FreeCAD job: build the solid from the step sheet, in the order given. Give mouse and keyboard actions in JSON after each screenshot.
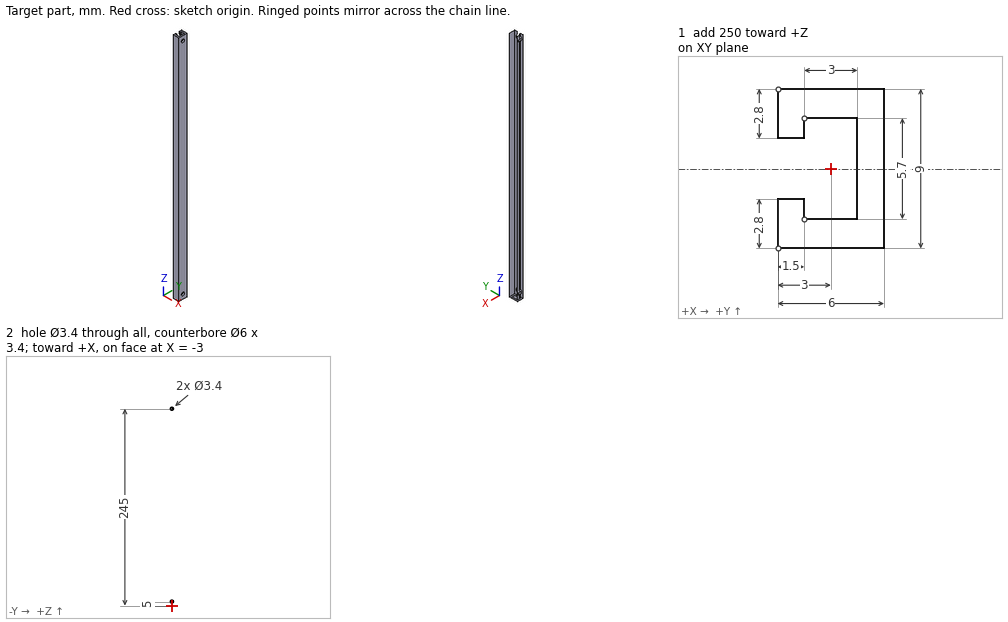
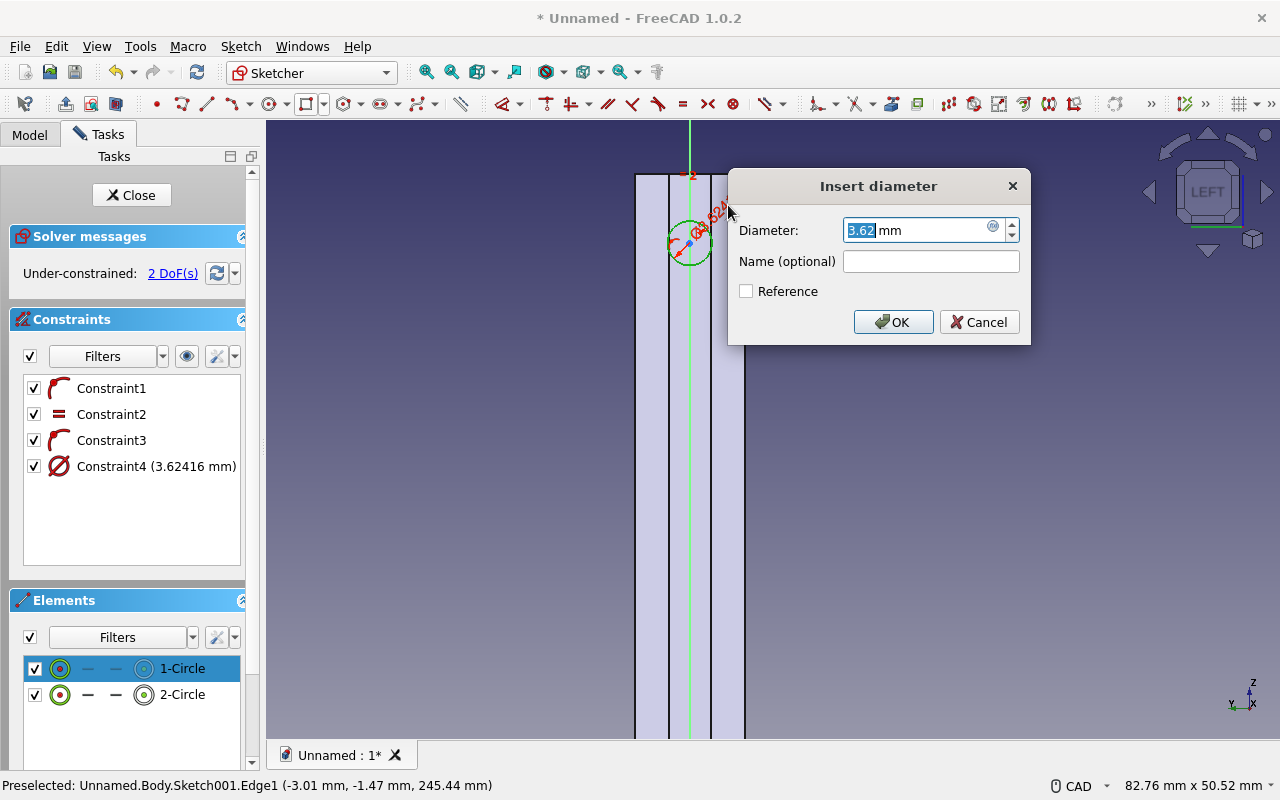
{"action": "type", "text": "3.4"}
{"action": "key", "text": "Return"}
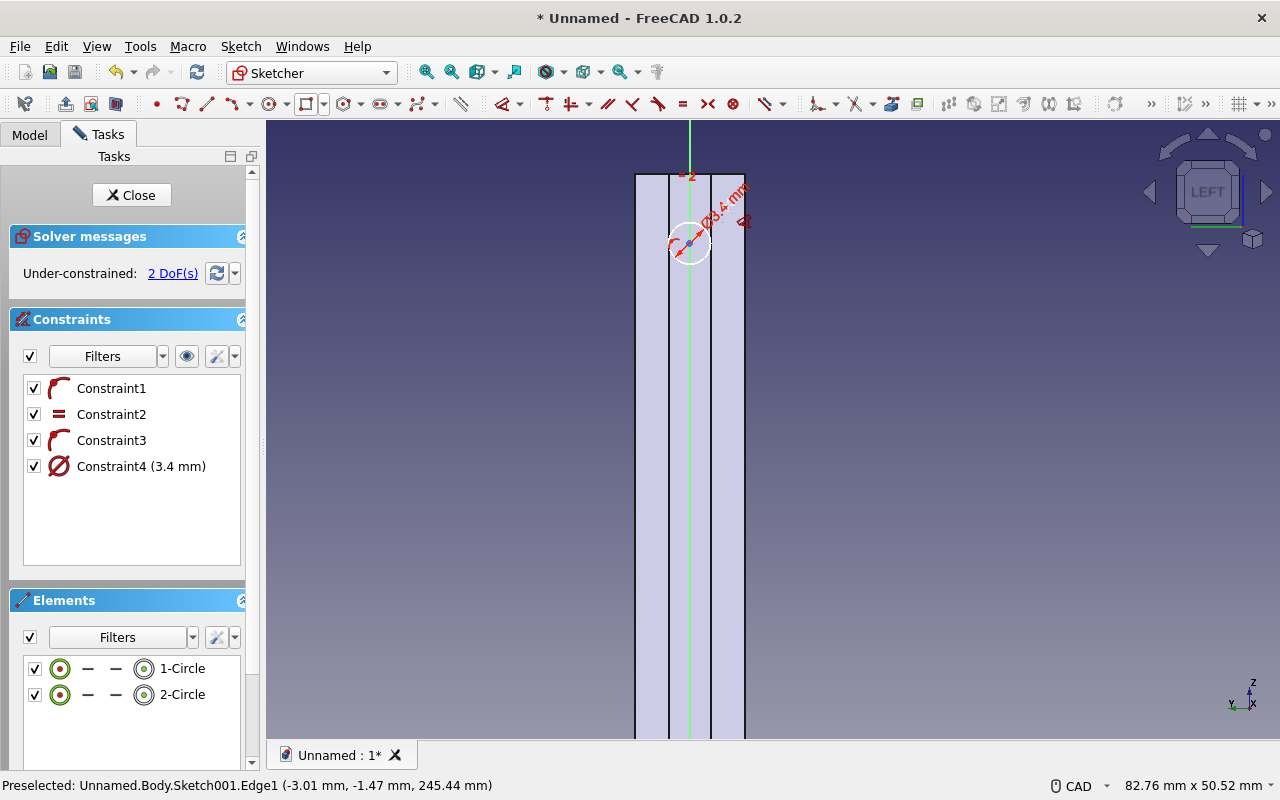
{"action": "scroll", "coordinate": [707, 227], "scroll_direction": "down", "scroll_amount": 10}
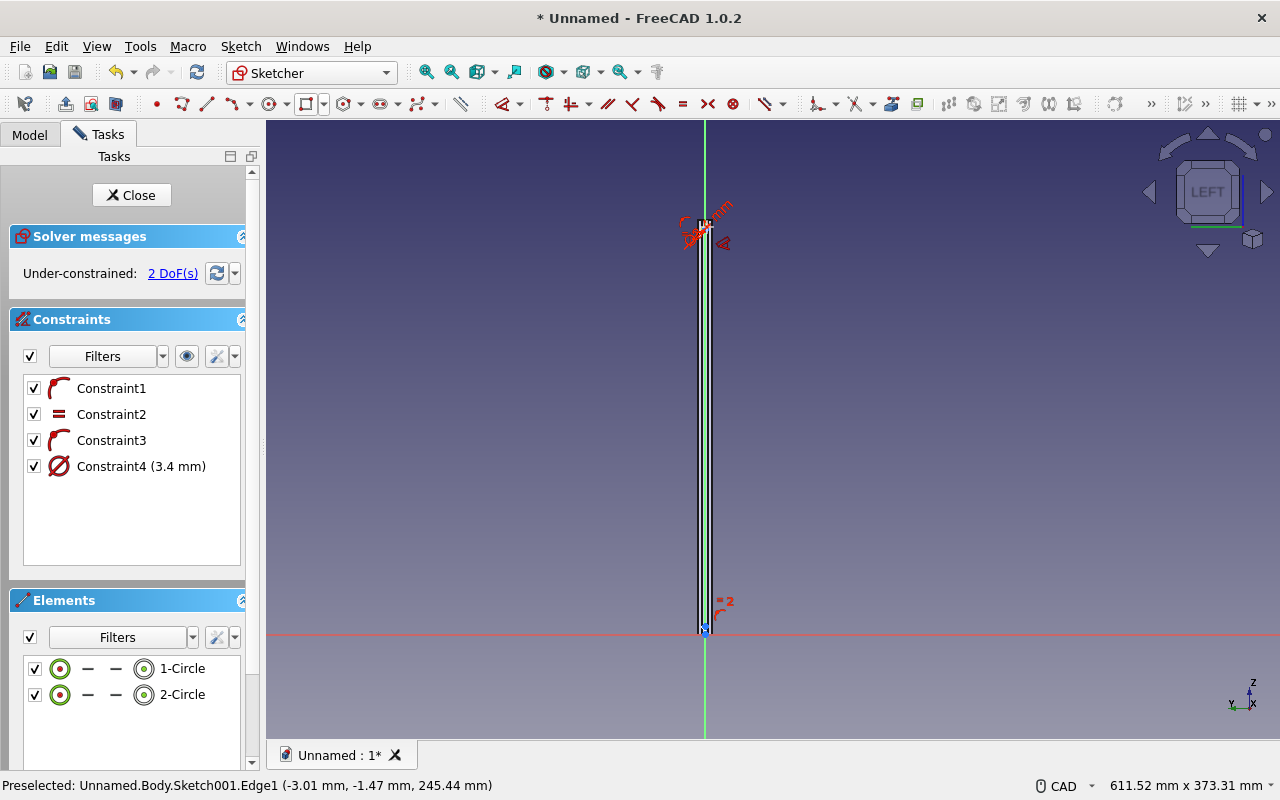
{"action": "scroll", "coordinate": [705, 627], "scroll_direction": "up", "scroll_amount": 8}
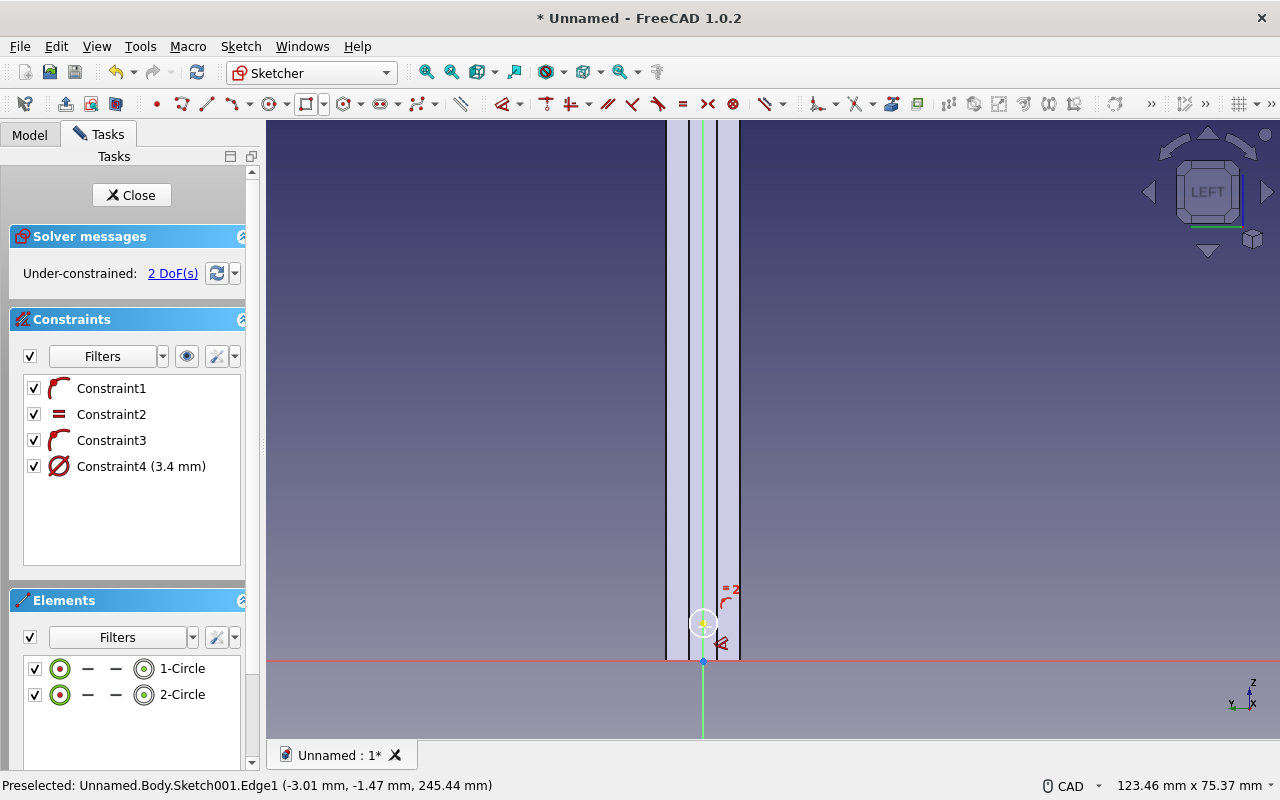
{"action": "left_click", "coordinate": [703, 623]}
{"action": "left_click", "coordinate": [737, 642]}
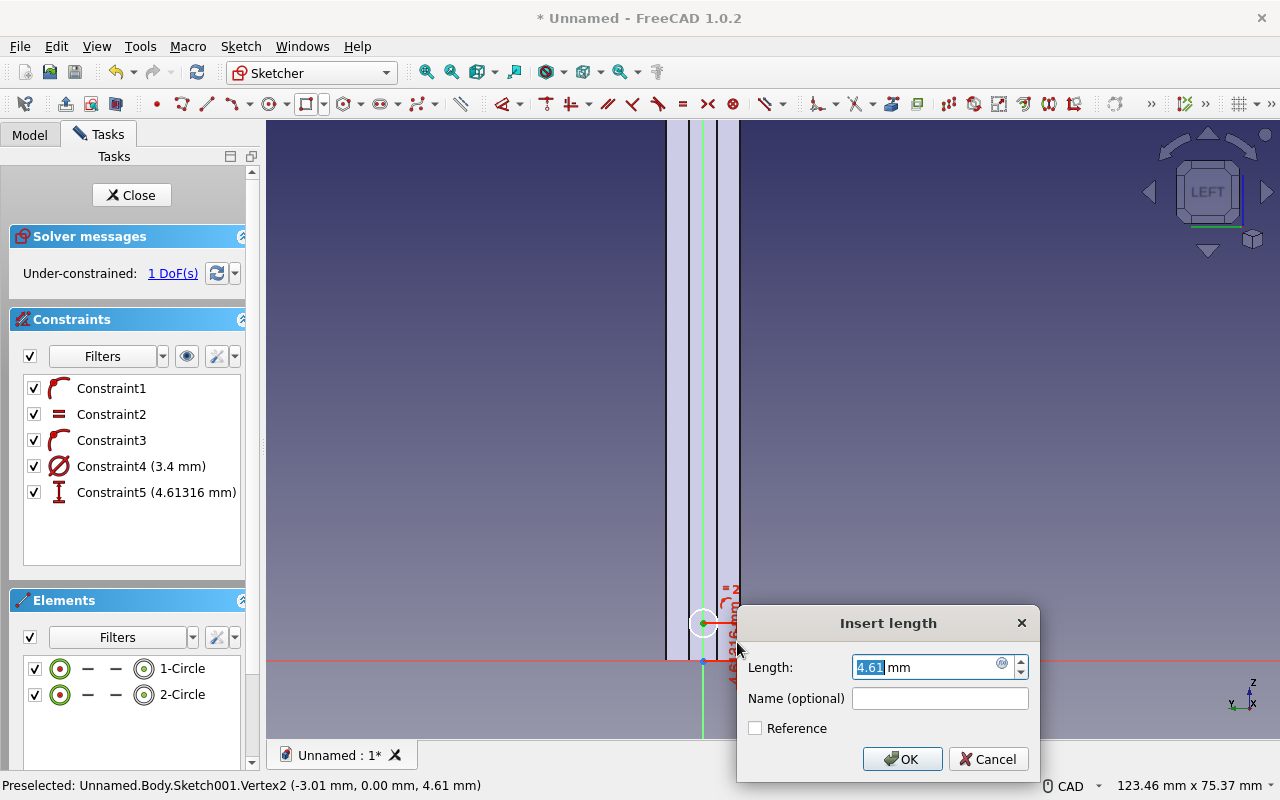
{"action": "type", "text": "5"}
{"action": "key", "text": "Return"}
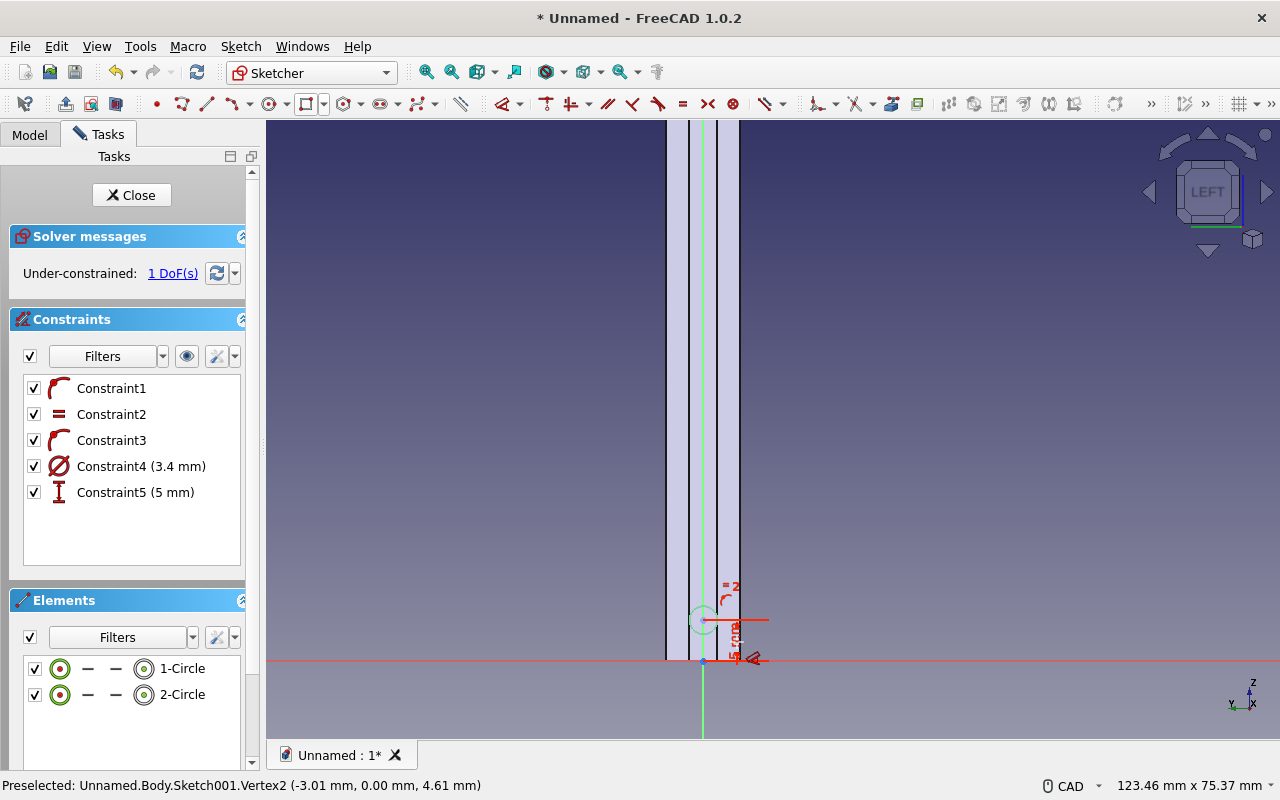
{"action": "scroll", "coordinate": [705, 627], "scroll_direction": "down", "scroll_amount": 8}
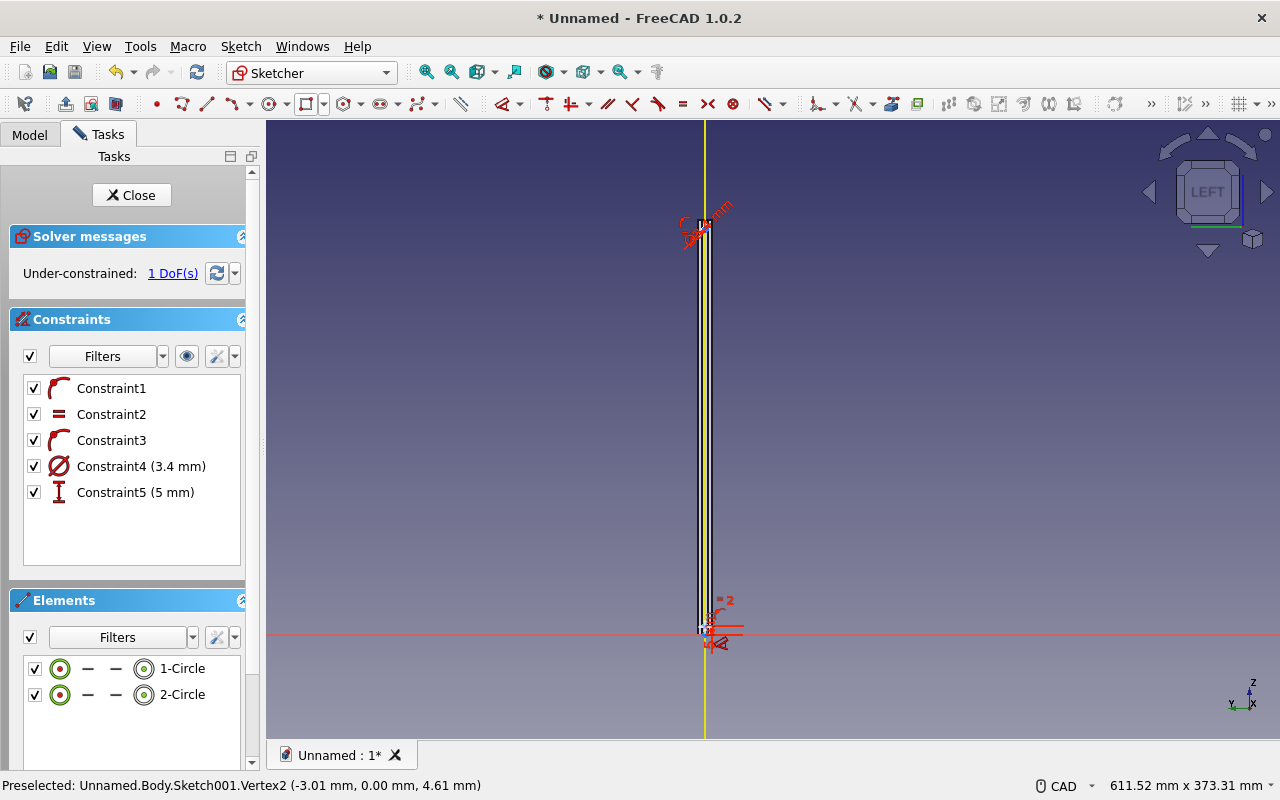
{"action": "left_click", "coordinate": [705, 229]}
{"action": "left_click", "coordinate": [739, 432]}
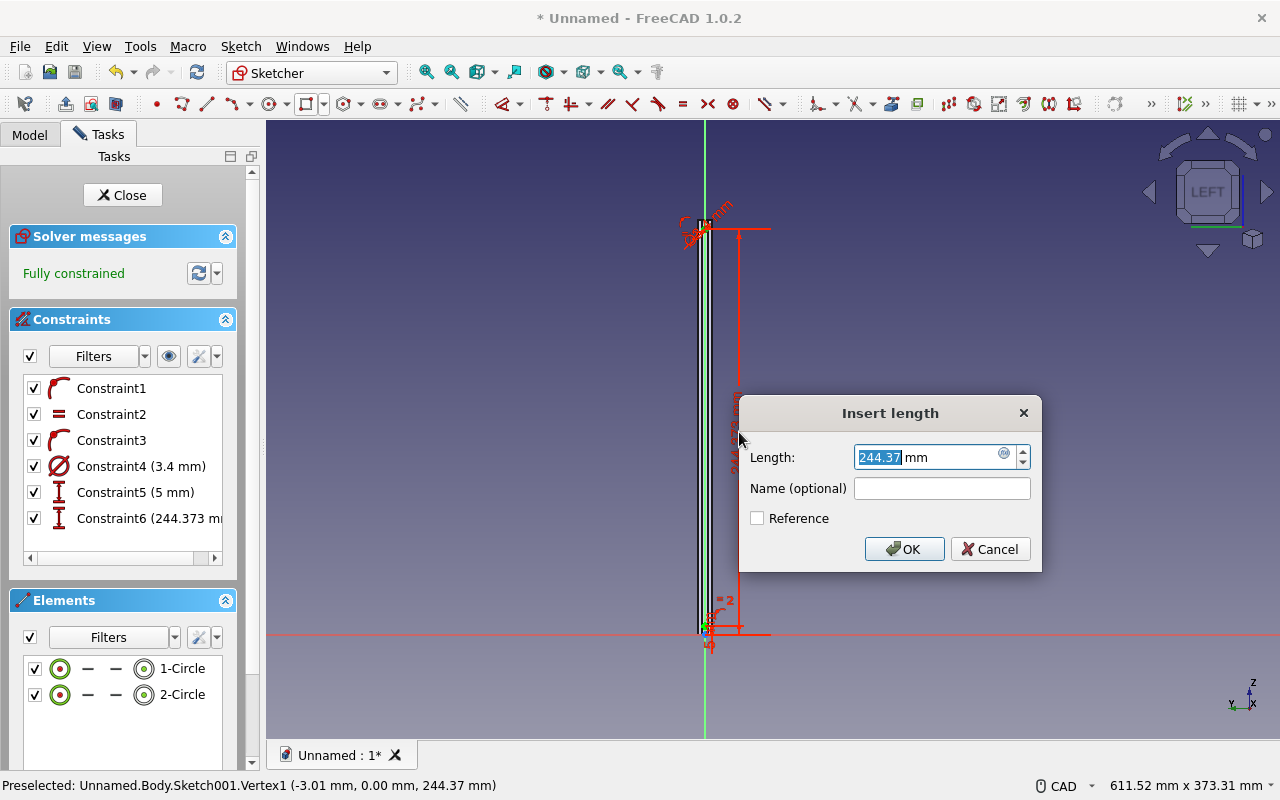
{"action": "type", "text": "245"}
{"action": "key", "text": "Return"}
{"action": "key", "text": "Escape"}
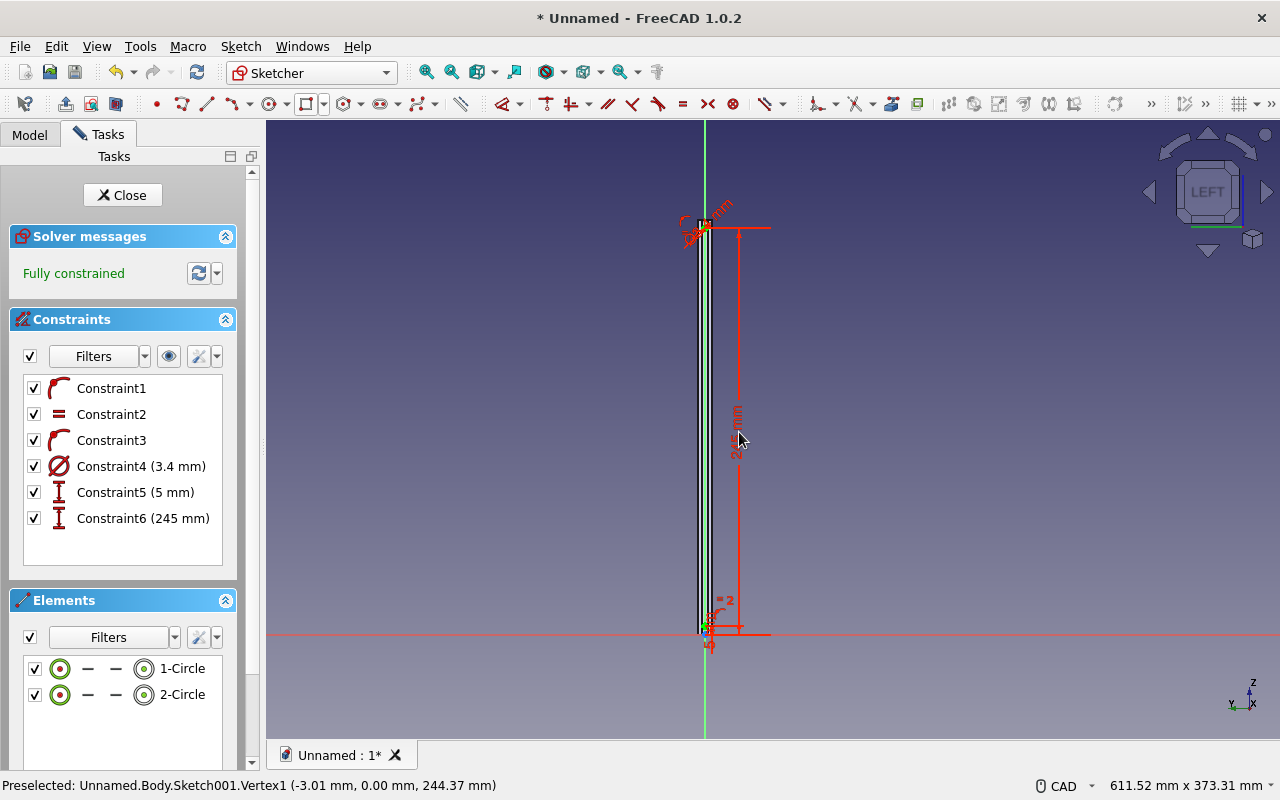
{"action": "left_click", "coordinate": [123, 195]}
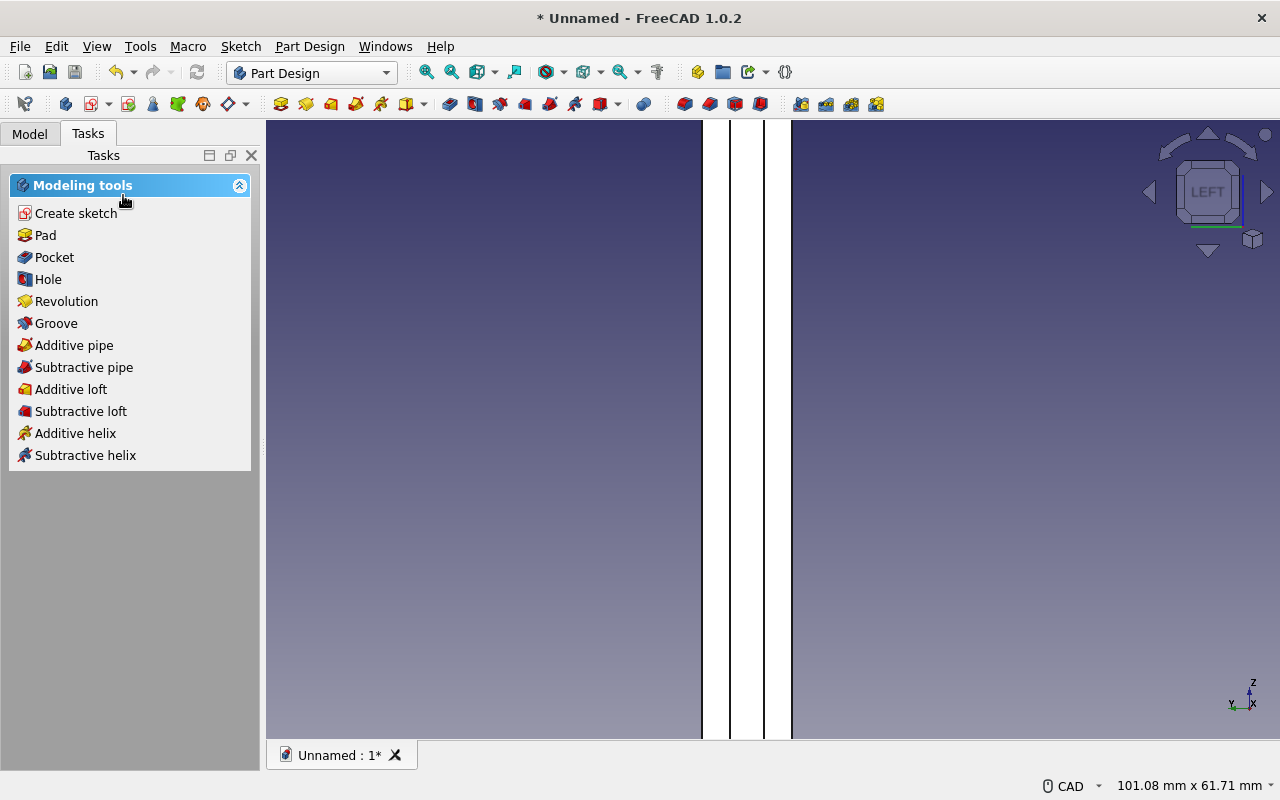
{"action": "left_click", "coordinate": [475, 104]}